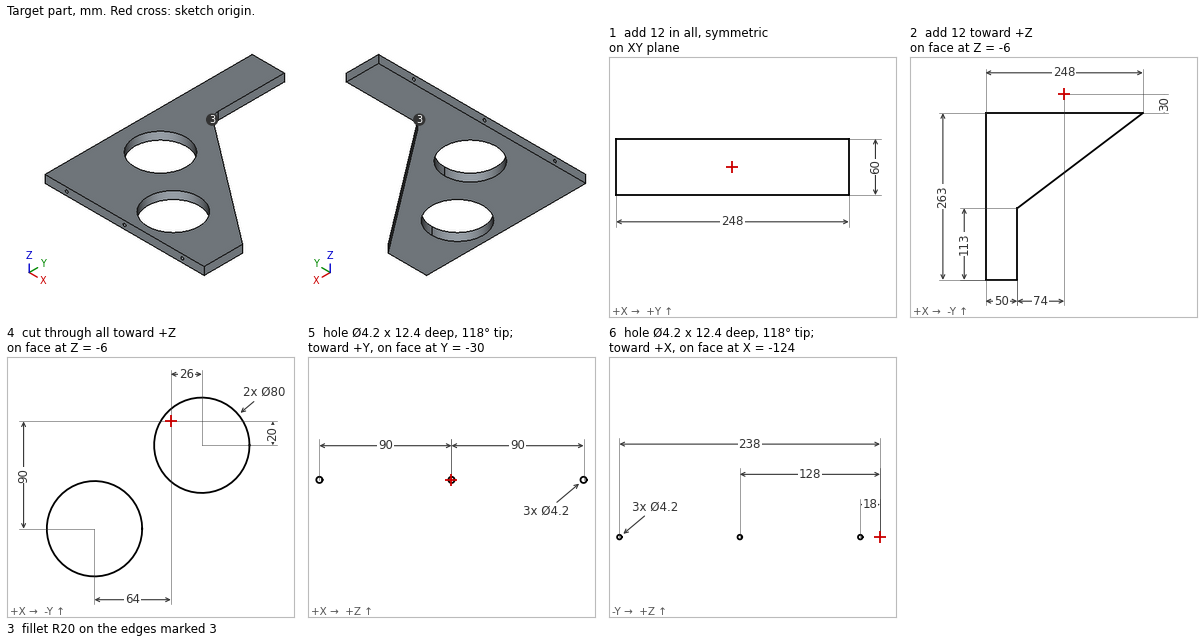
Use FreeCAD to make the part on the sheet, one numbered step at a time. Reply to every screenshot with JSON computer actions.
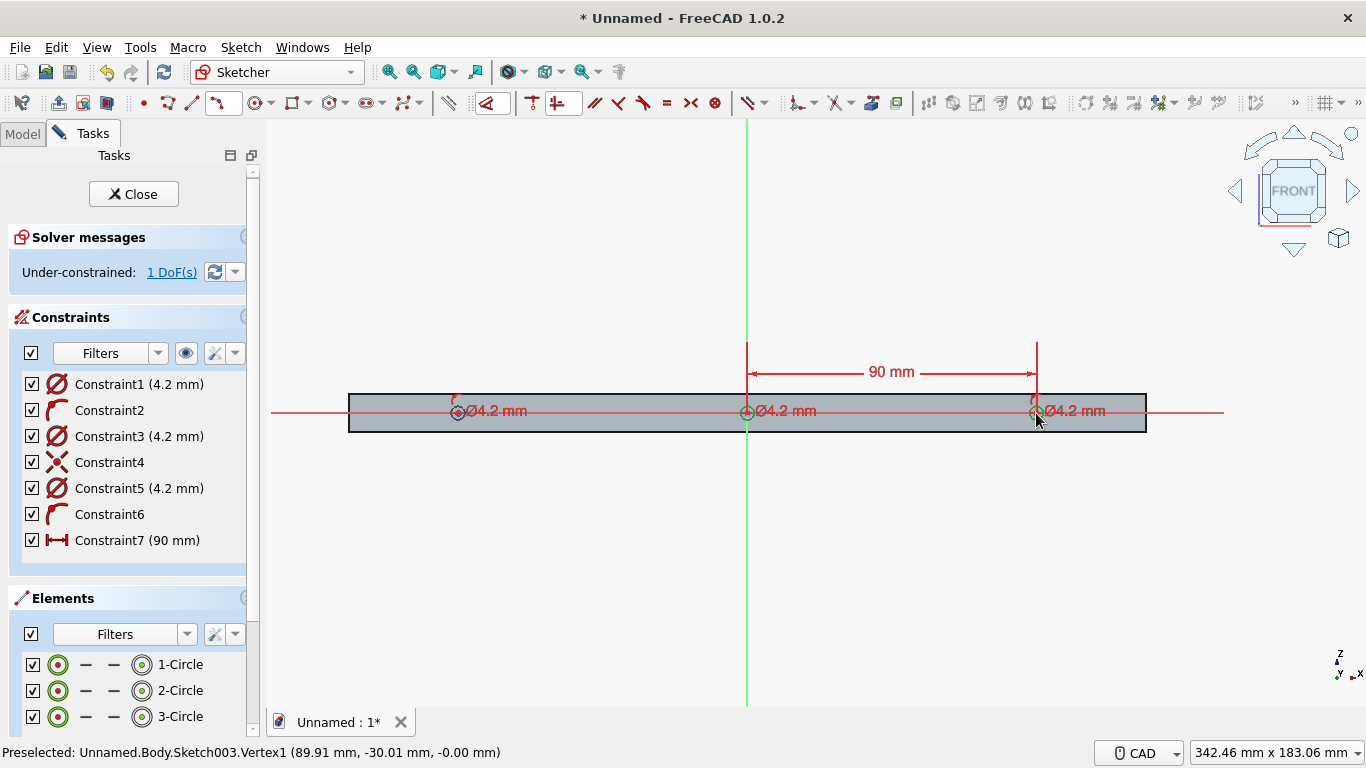
{"action": "left_click", "coordinate": [458, 413]}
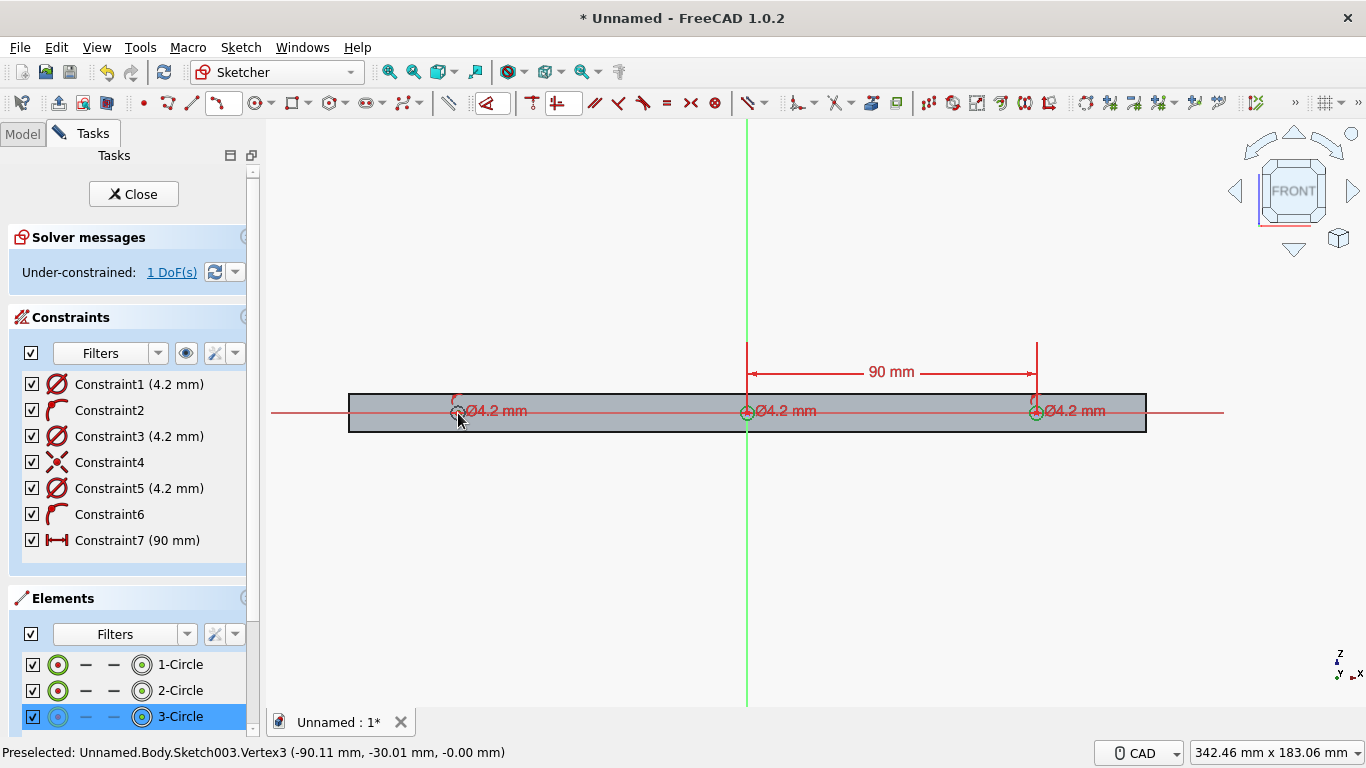
{"action": "key", "text": "l"}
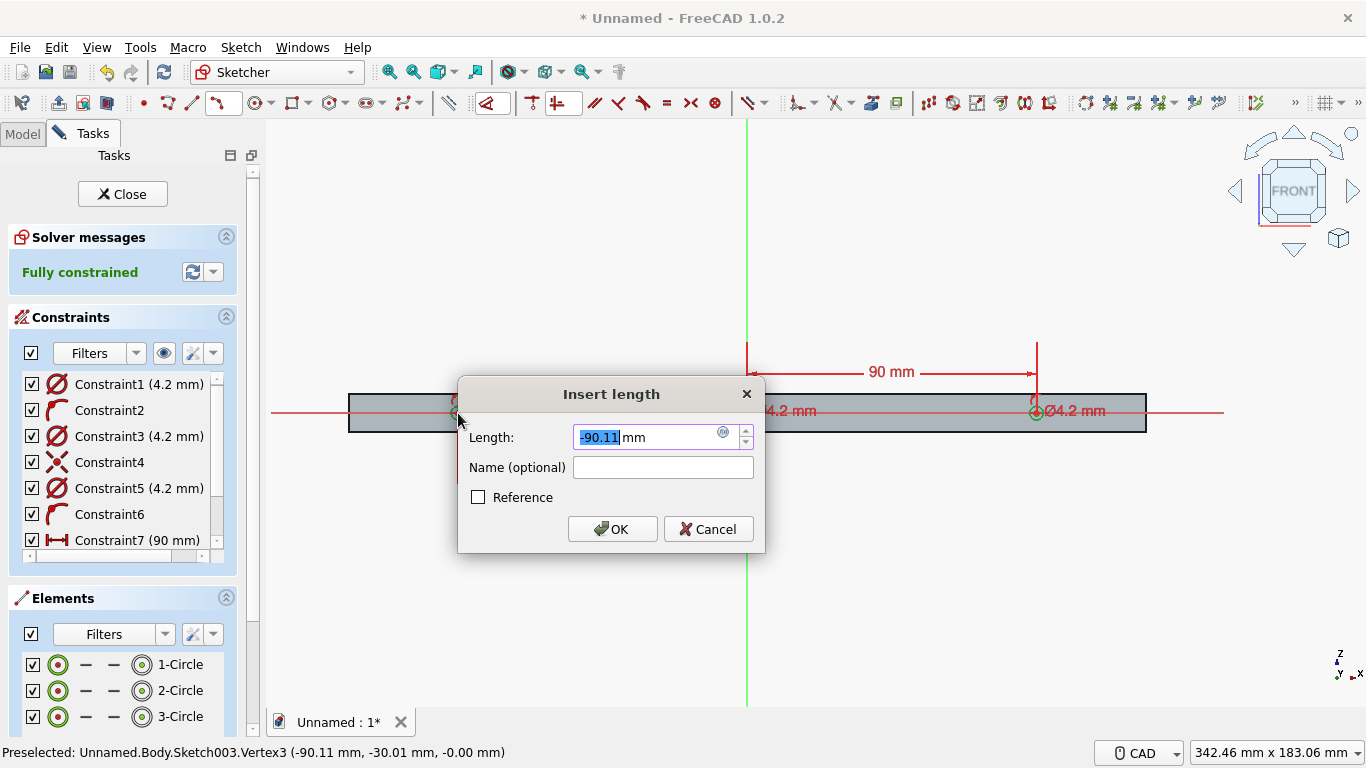
{"action": "type", "text": "-90"}
{"action": "key", "text": "Return"}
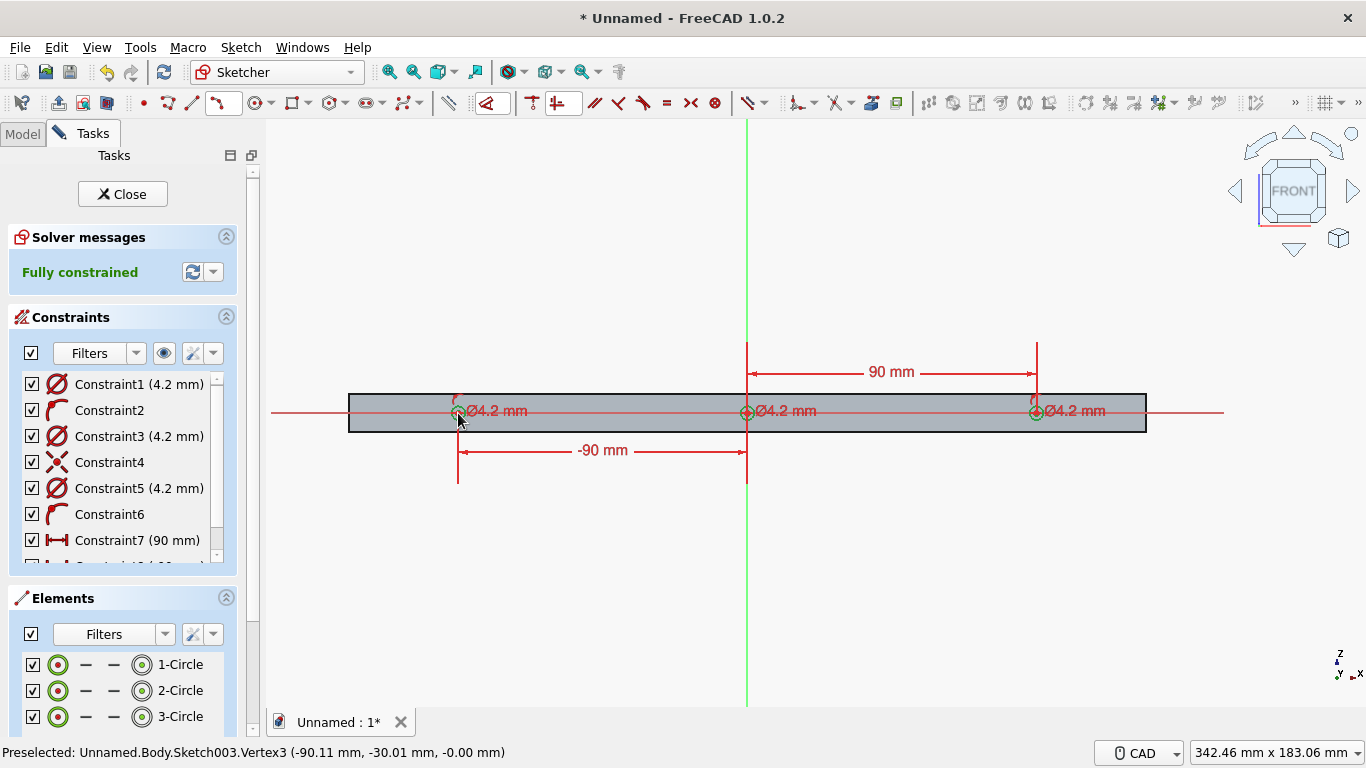
{"action": "left_click", "coordinate": [123, 194]}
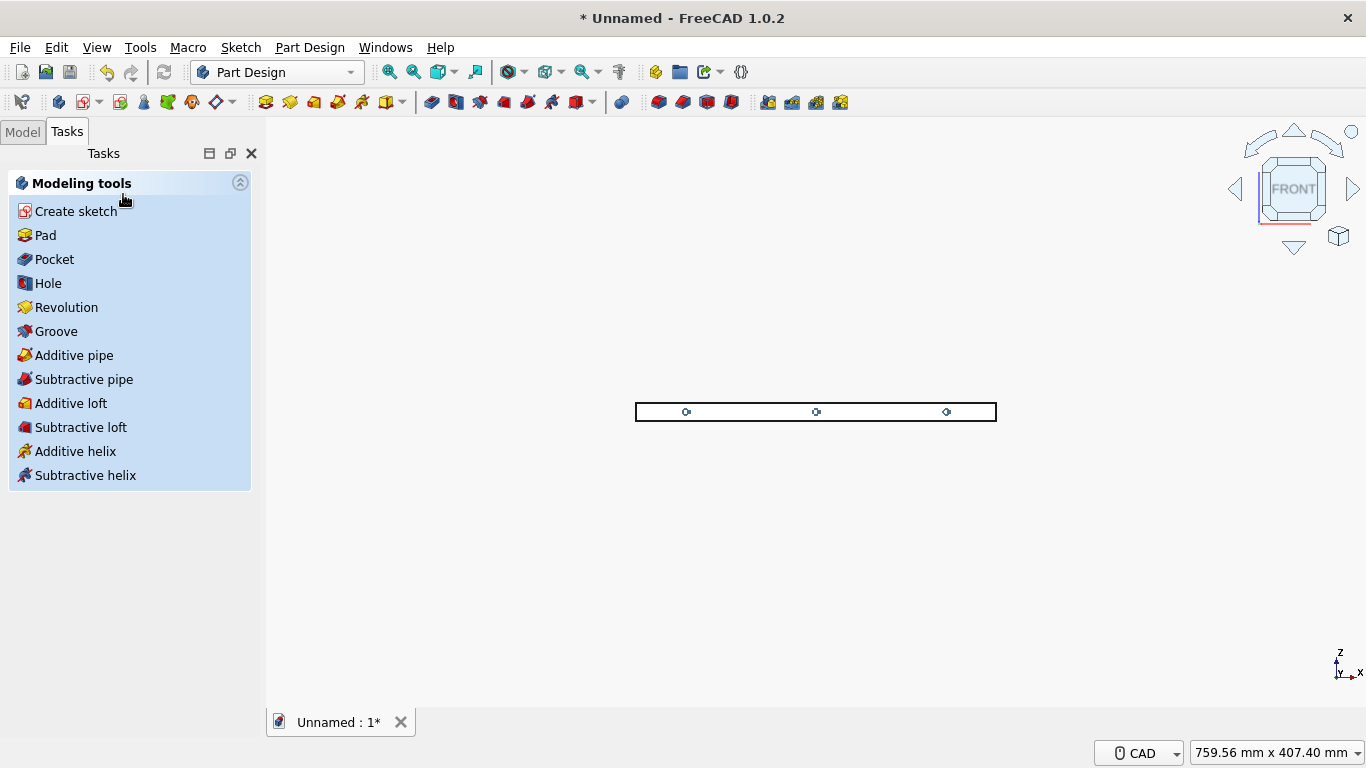
{"action": "left_click", "coordinate": [456, 102]}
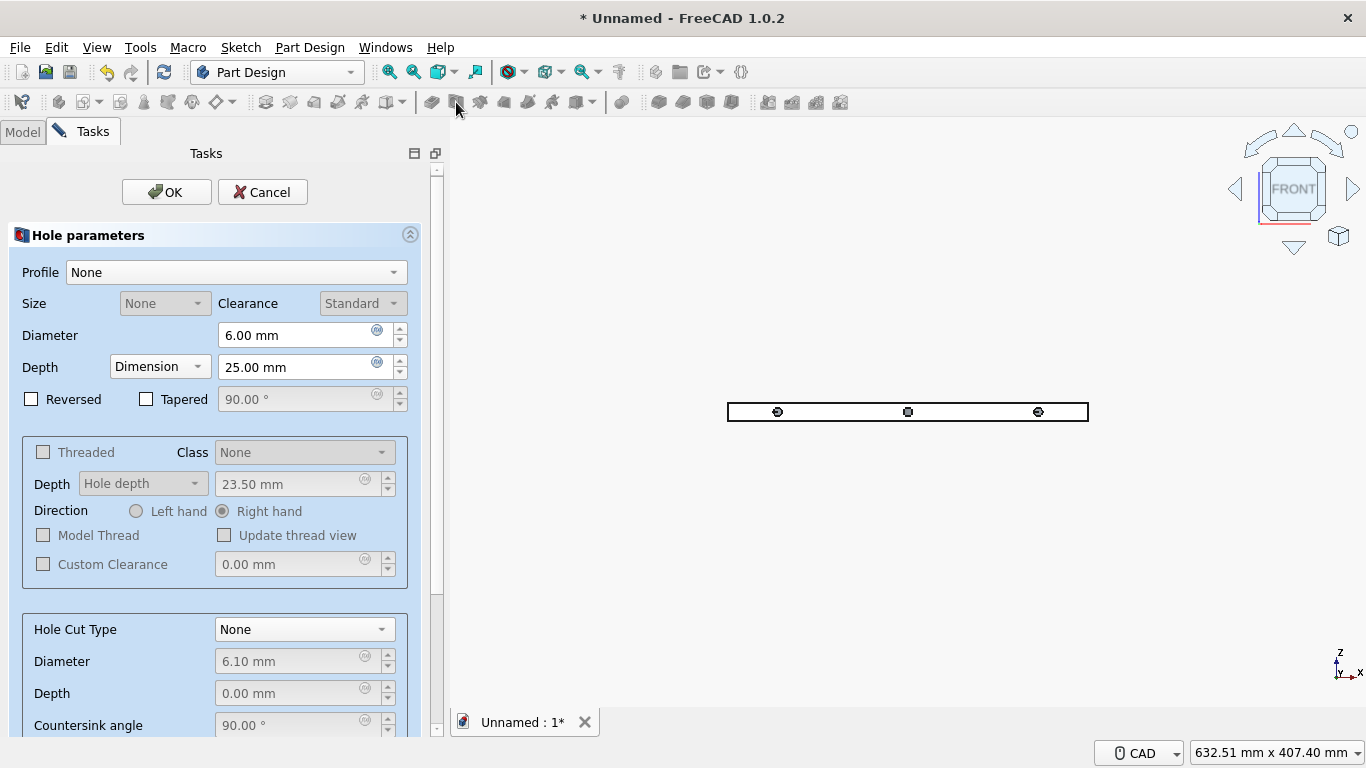
{"action": "triple_click", "coordinate": [305, 335]}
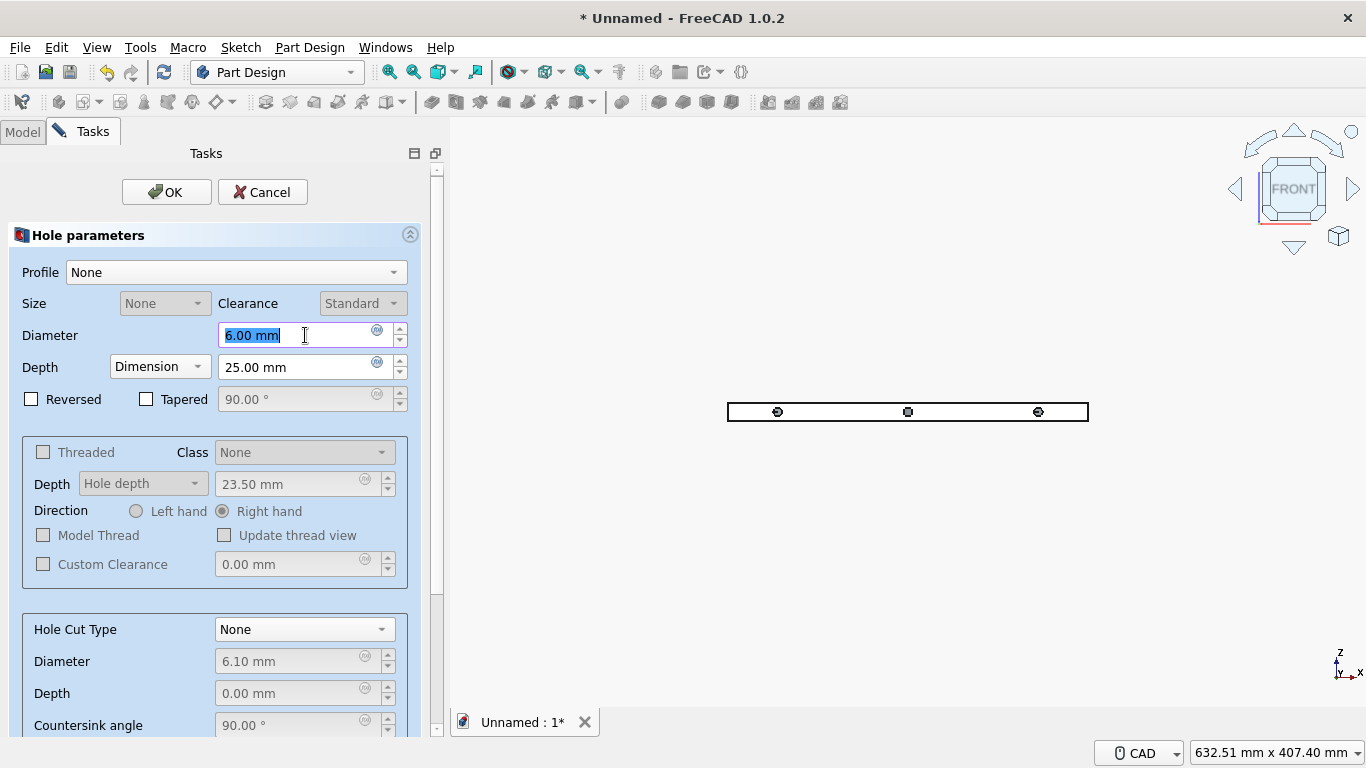
{"action": "type", "text": "4.2"}
{"action": "key", "text": "Tab"}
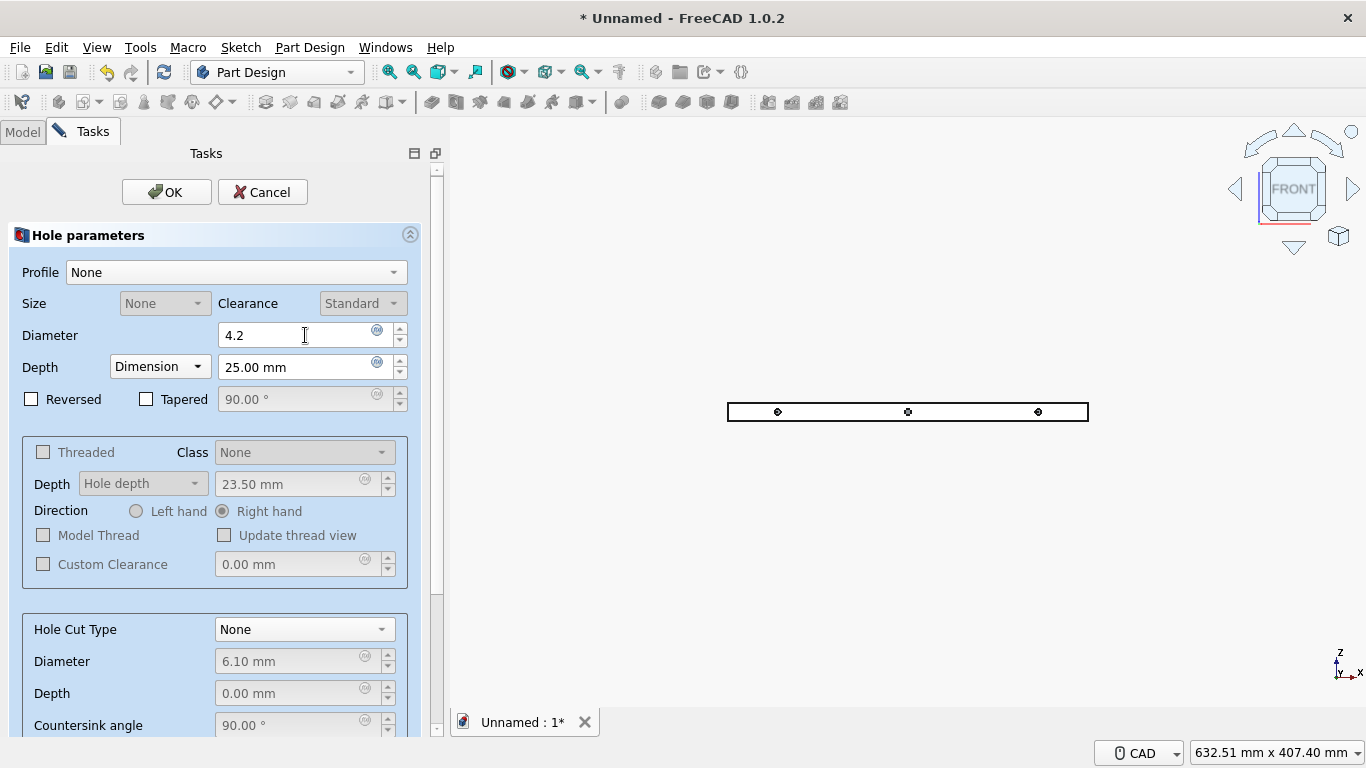
{"action": "triple_click", "coordinate": [305, 367]}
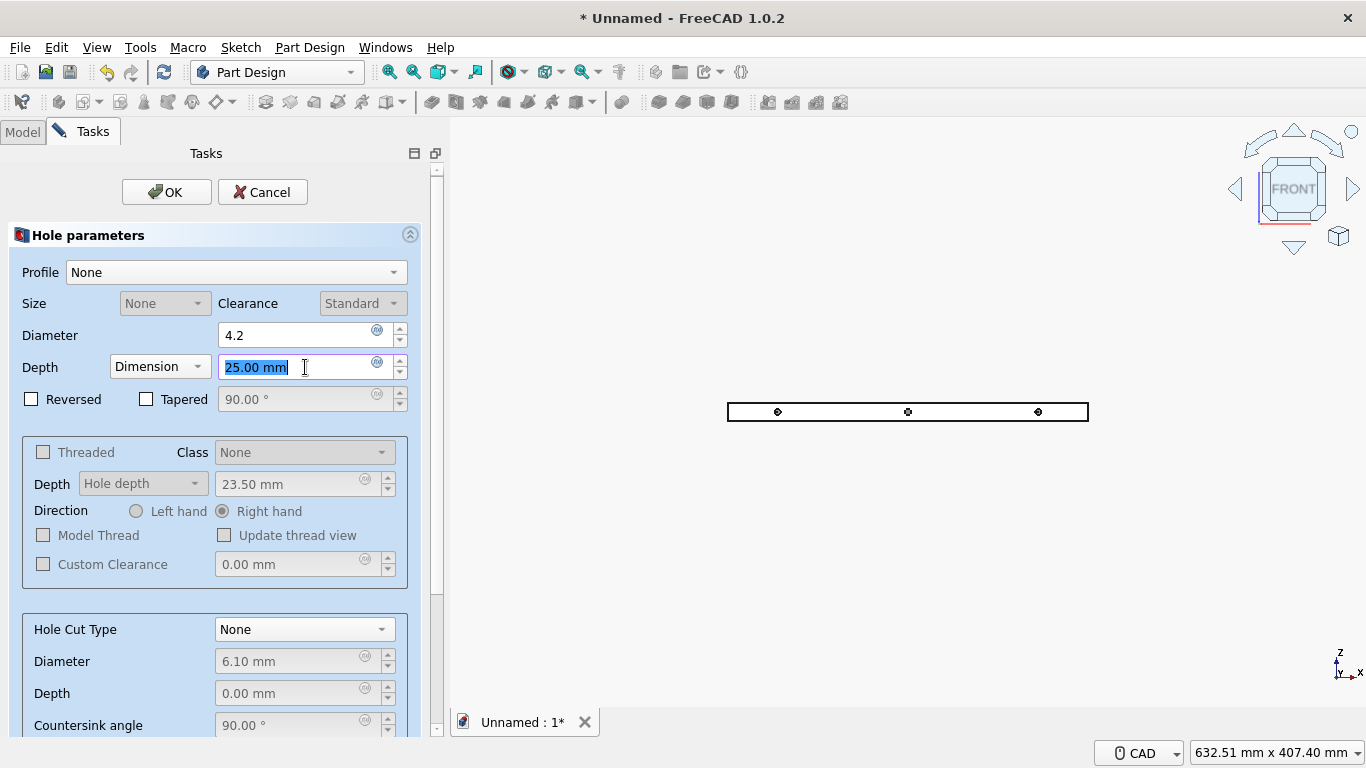
{"action": "type", "text": "12.4"}
{"action": "key", "text": "Tab"}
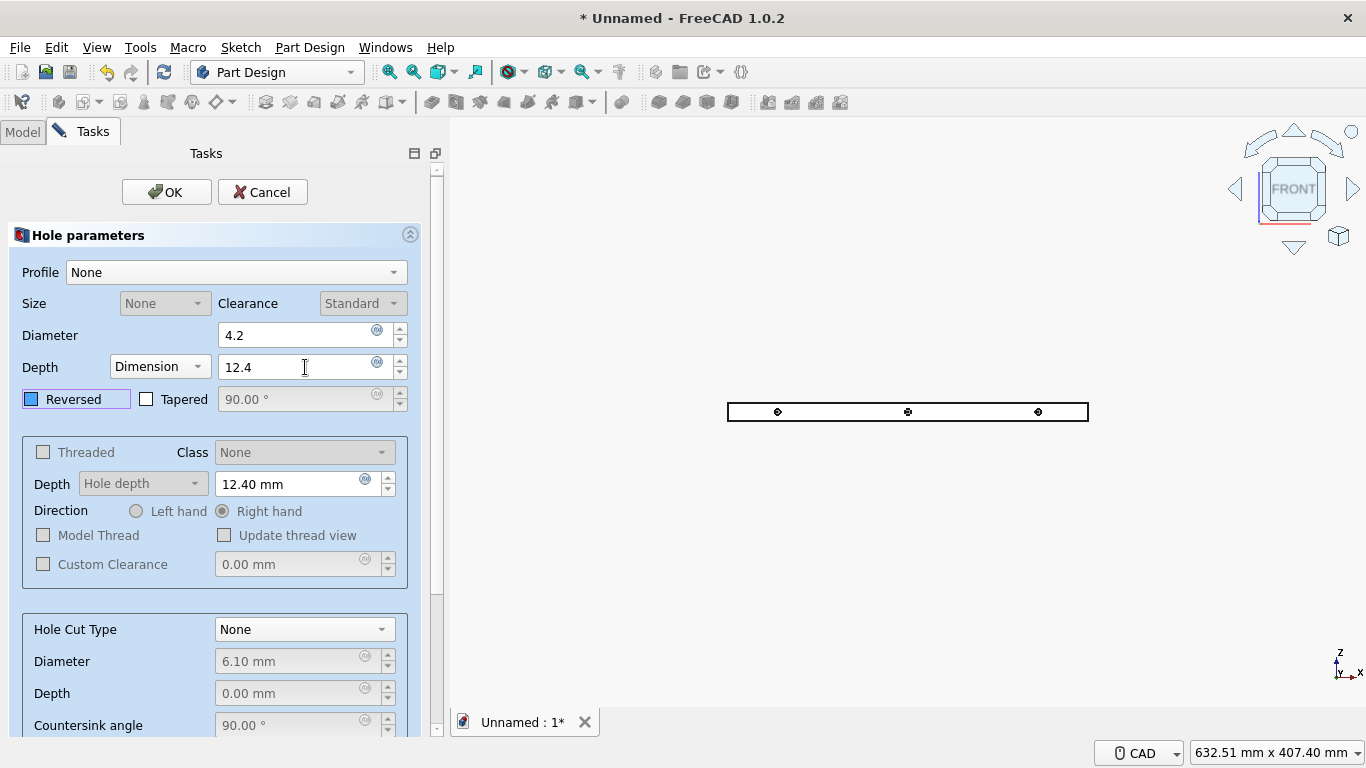
{"action": "left_click", "coordinate": [167, 192]}